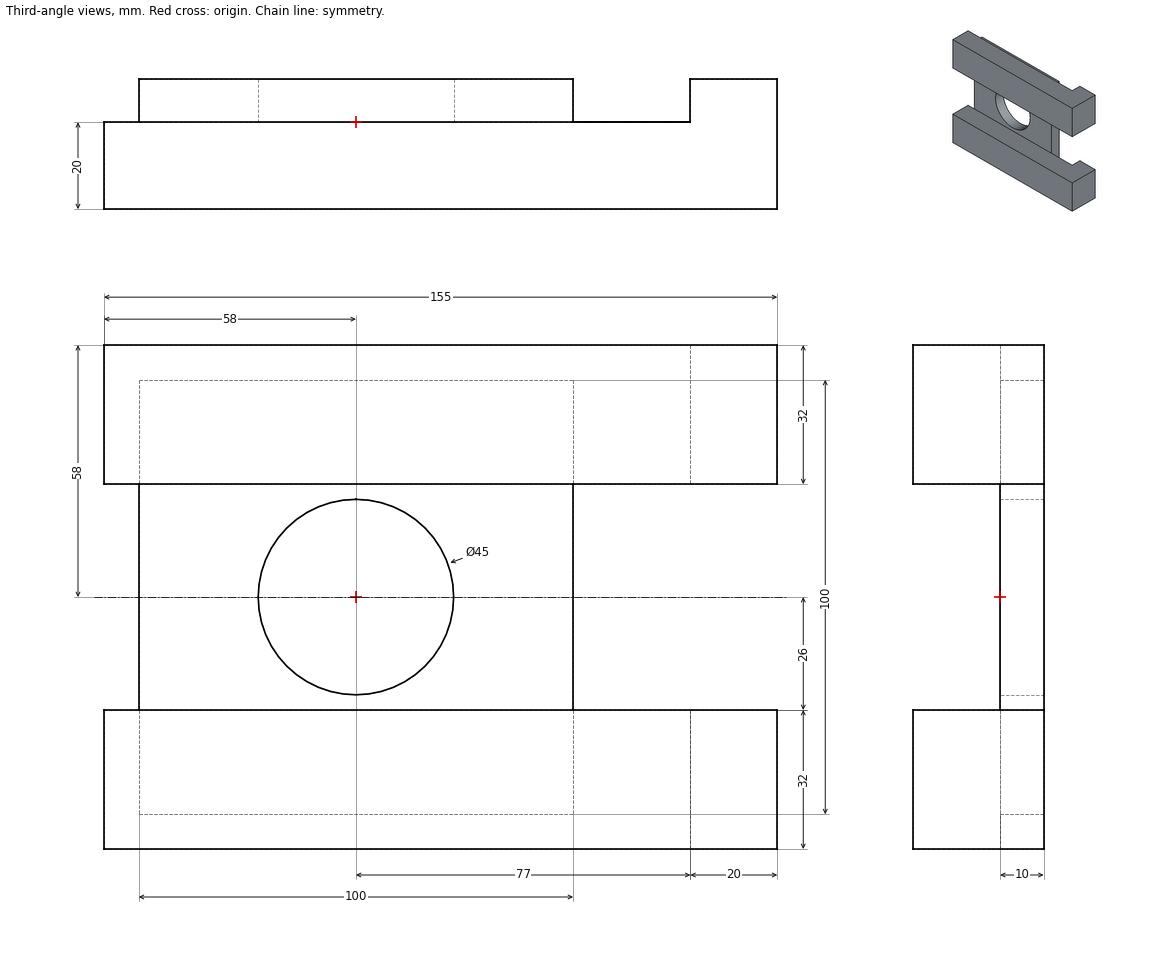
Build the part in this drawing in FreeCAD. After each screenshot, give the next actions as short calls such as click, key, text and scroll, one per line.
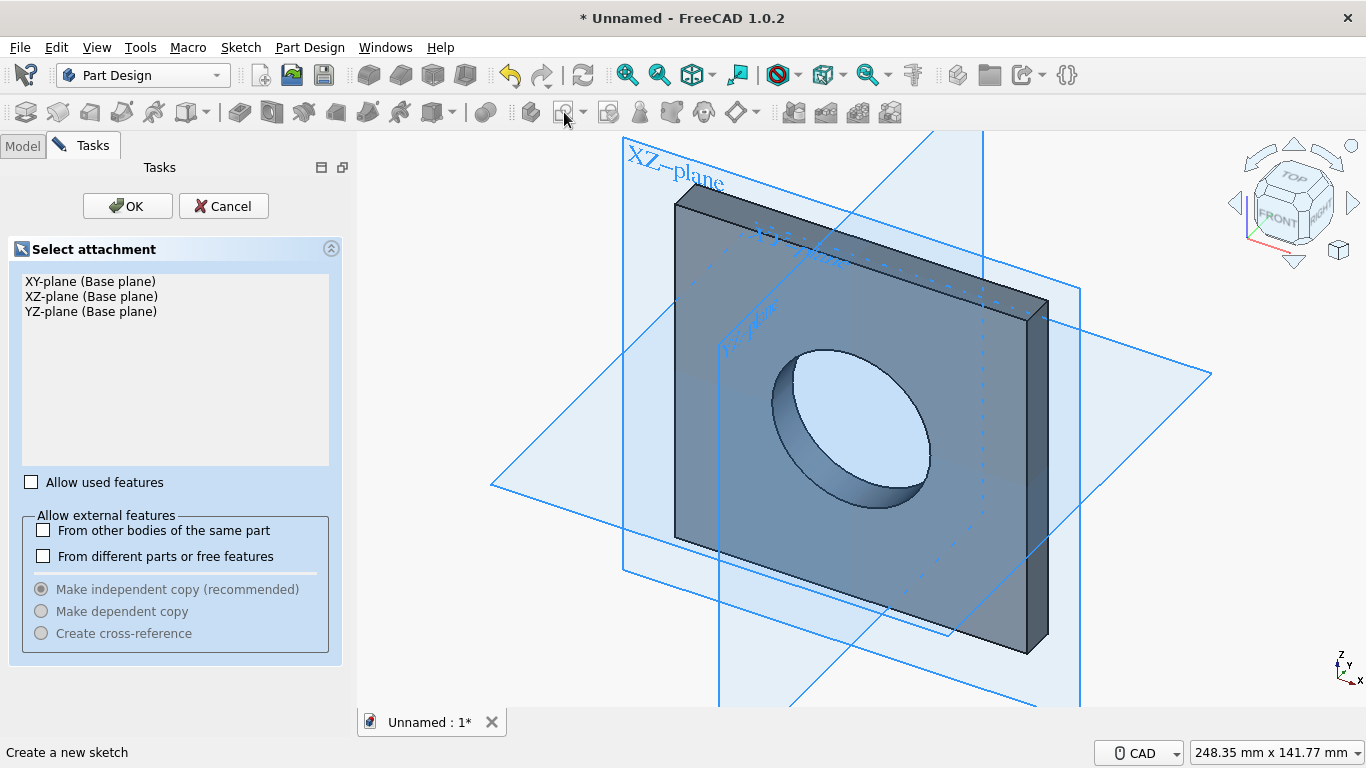
click(82, 296)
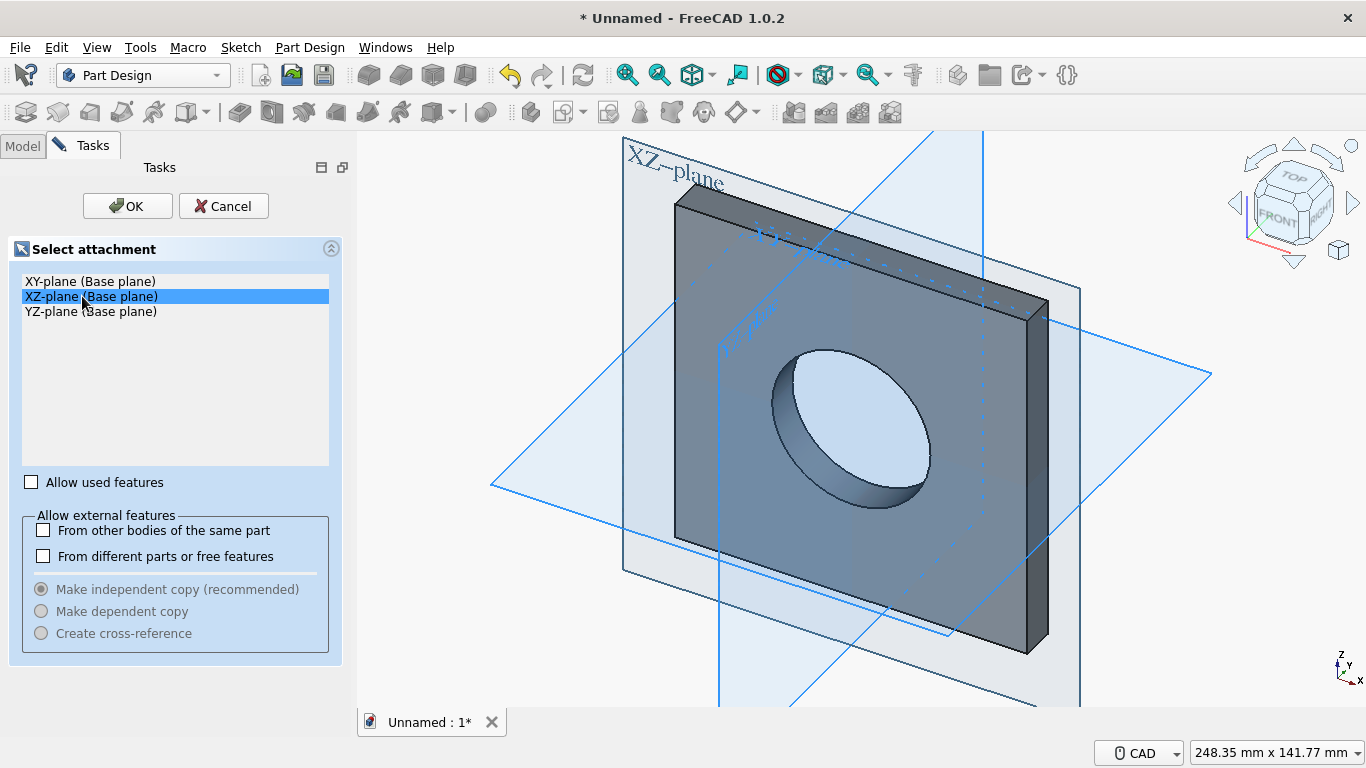
click(128, 206)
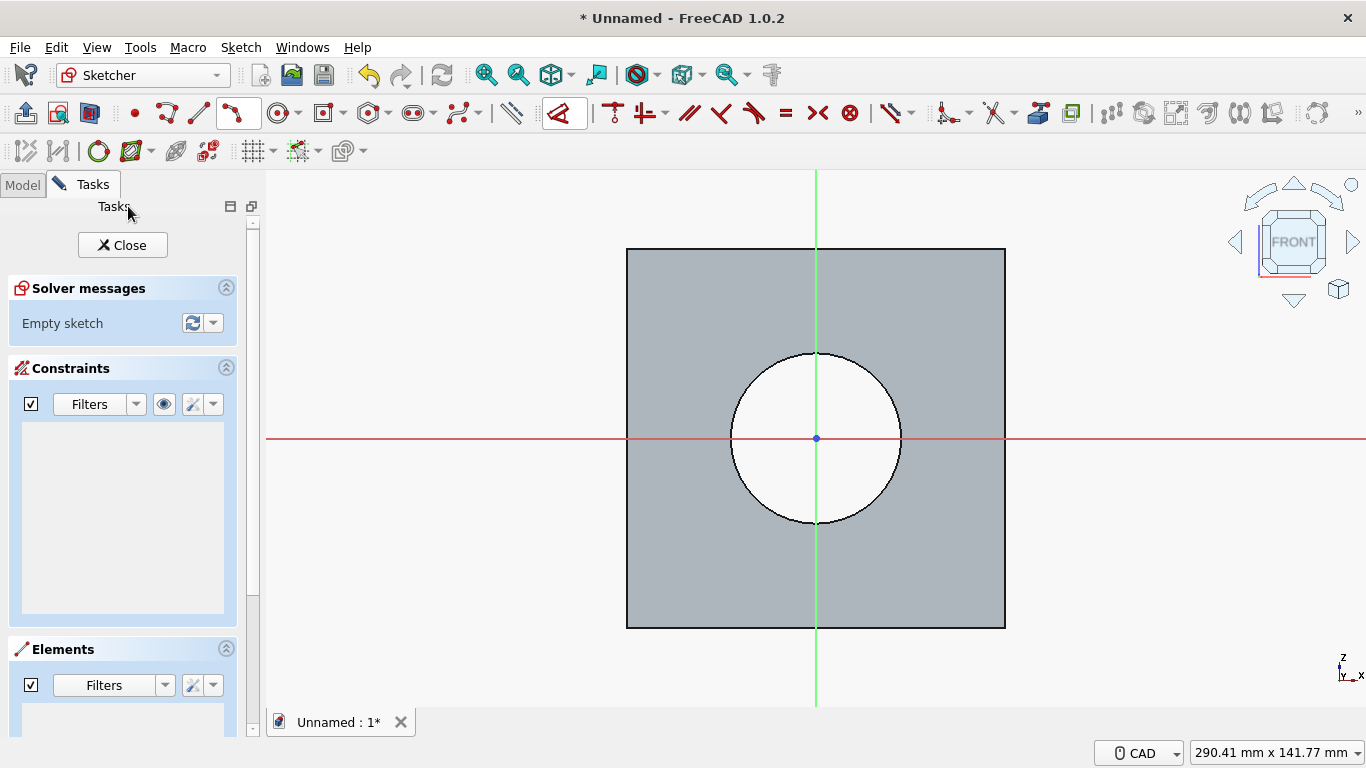
scroll(294, 439, down, 1)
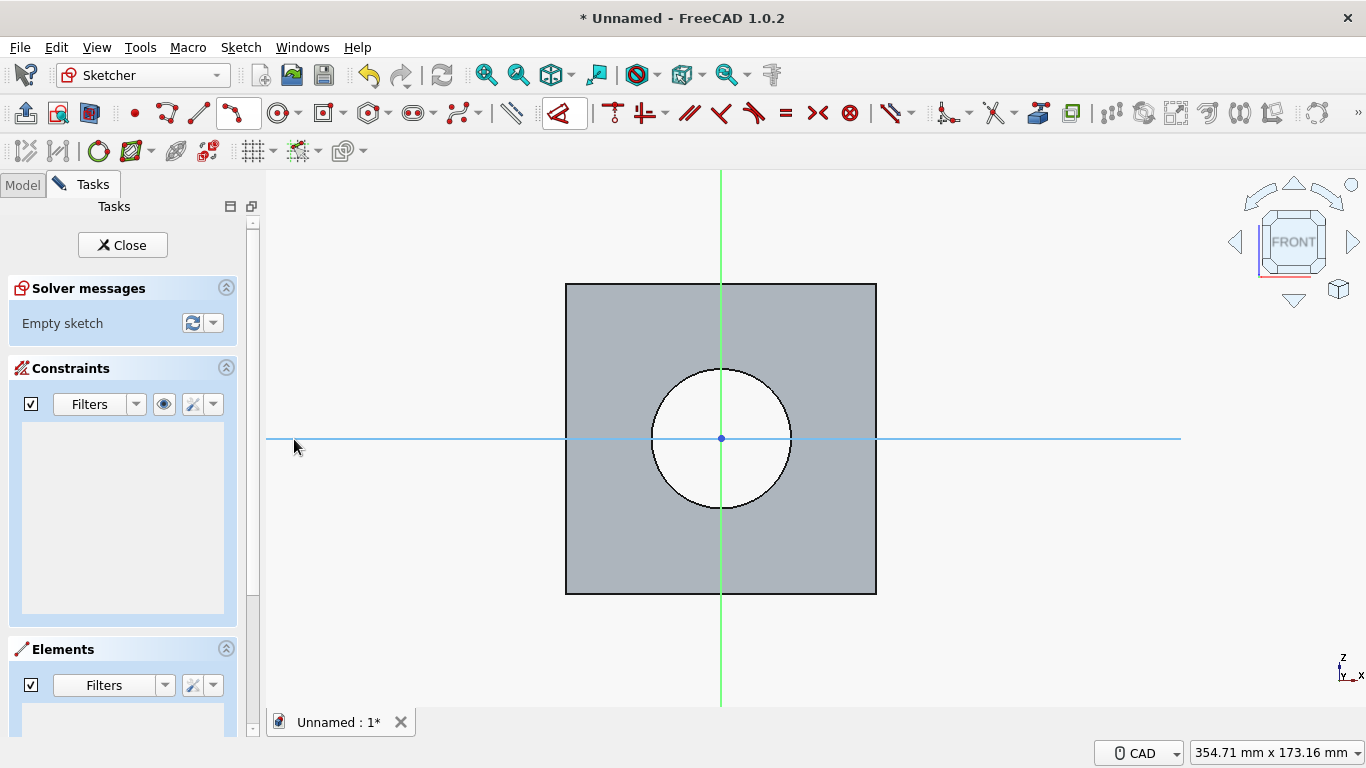
key(g)
key(r)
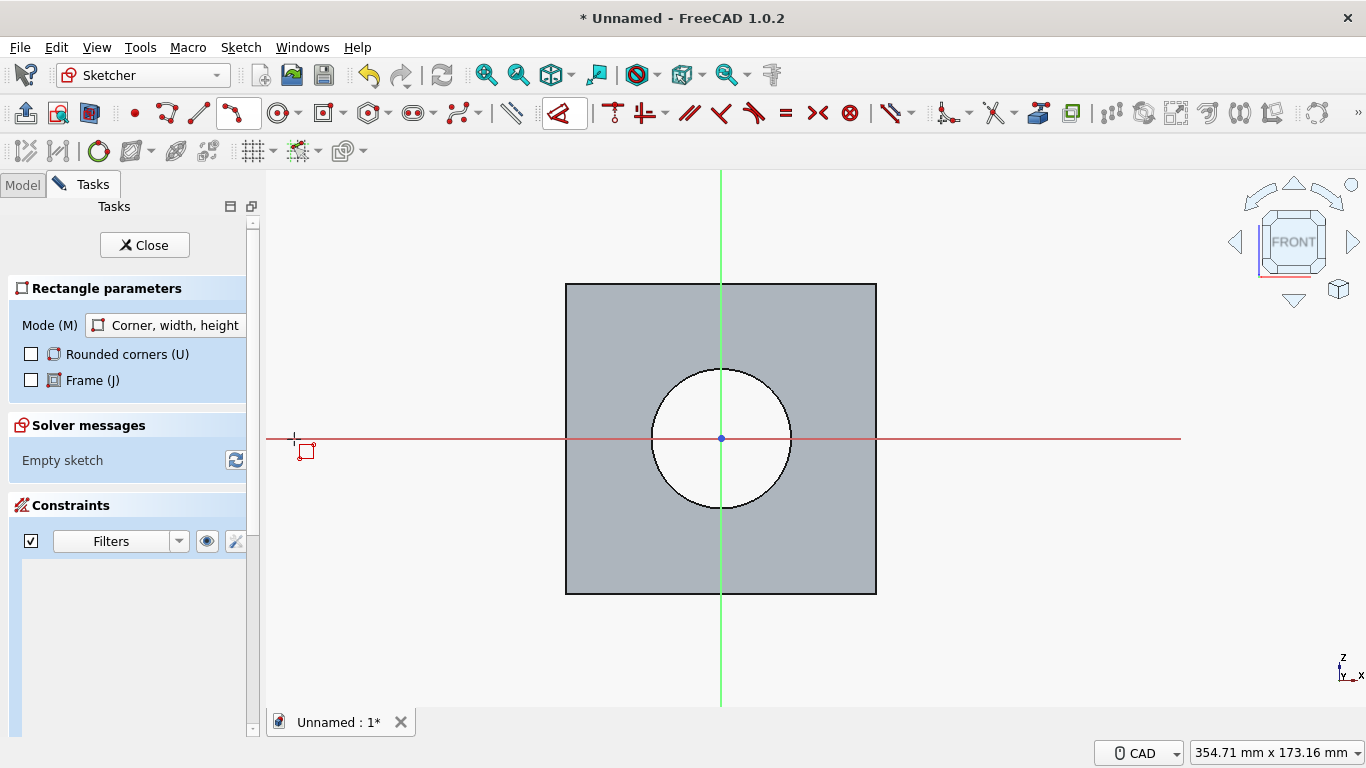
click(542, 259)
move(1022, 358)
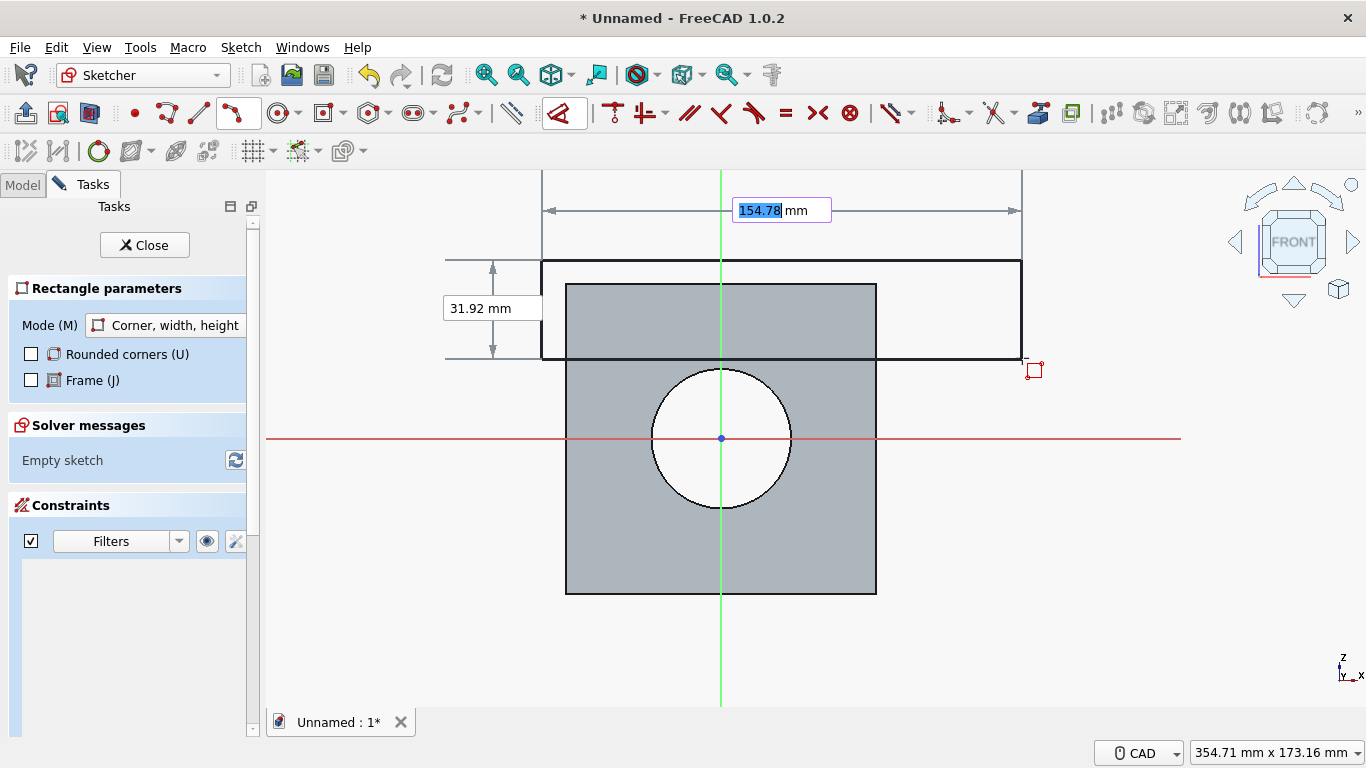
text(155)
key(Tab)
text(32)
key(Return)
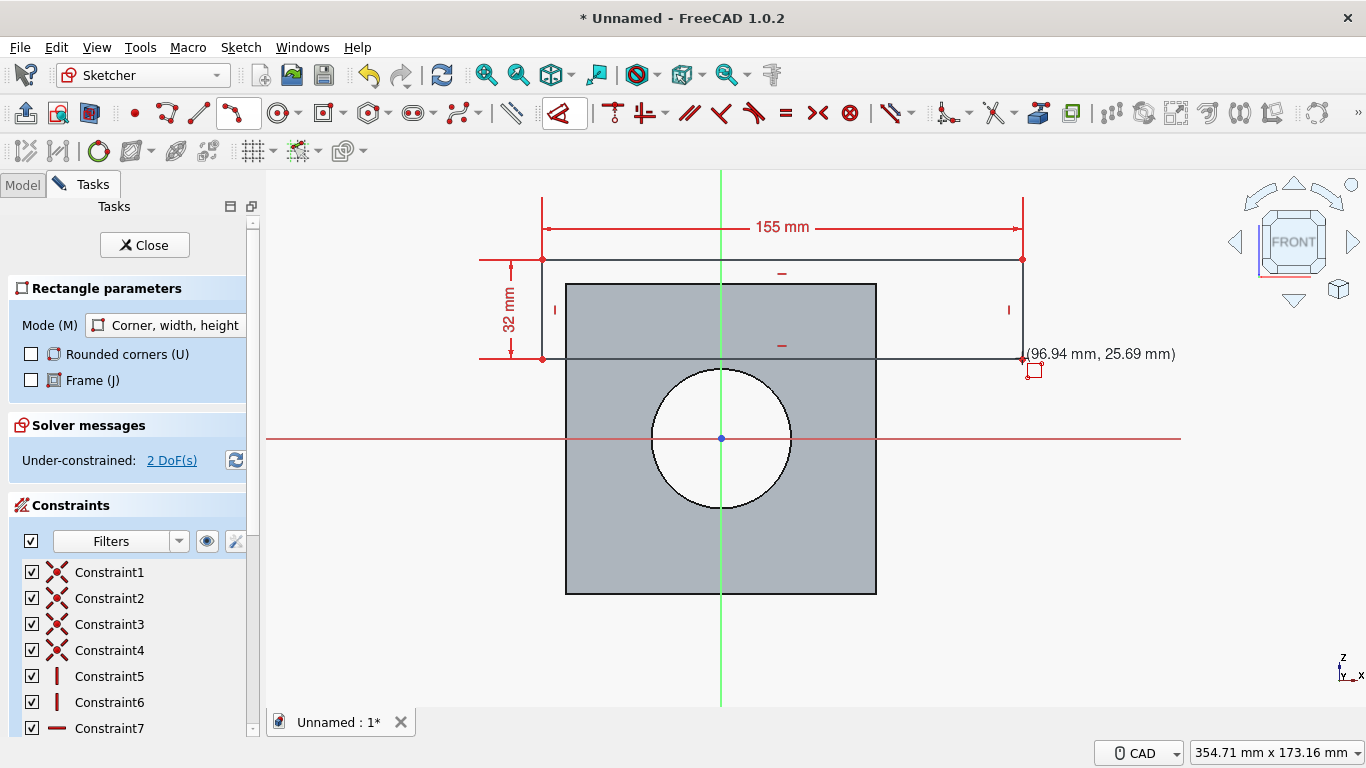
click(542, 519)
move(1022, 619)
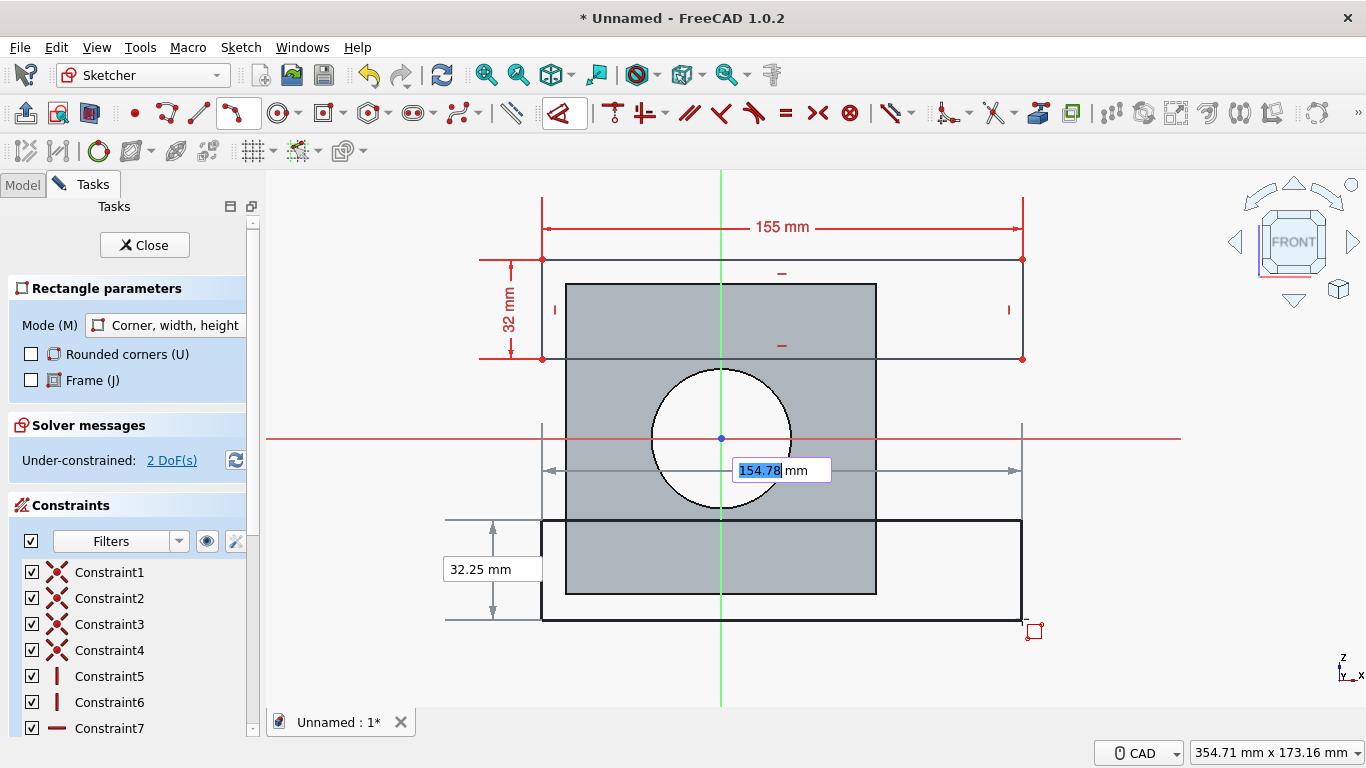
text(155)
key(Tab)
text(32)
key(Return)
key(Escape)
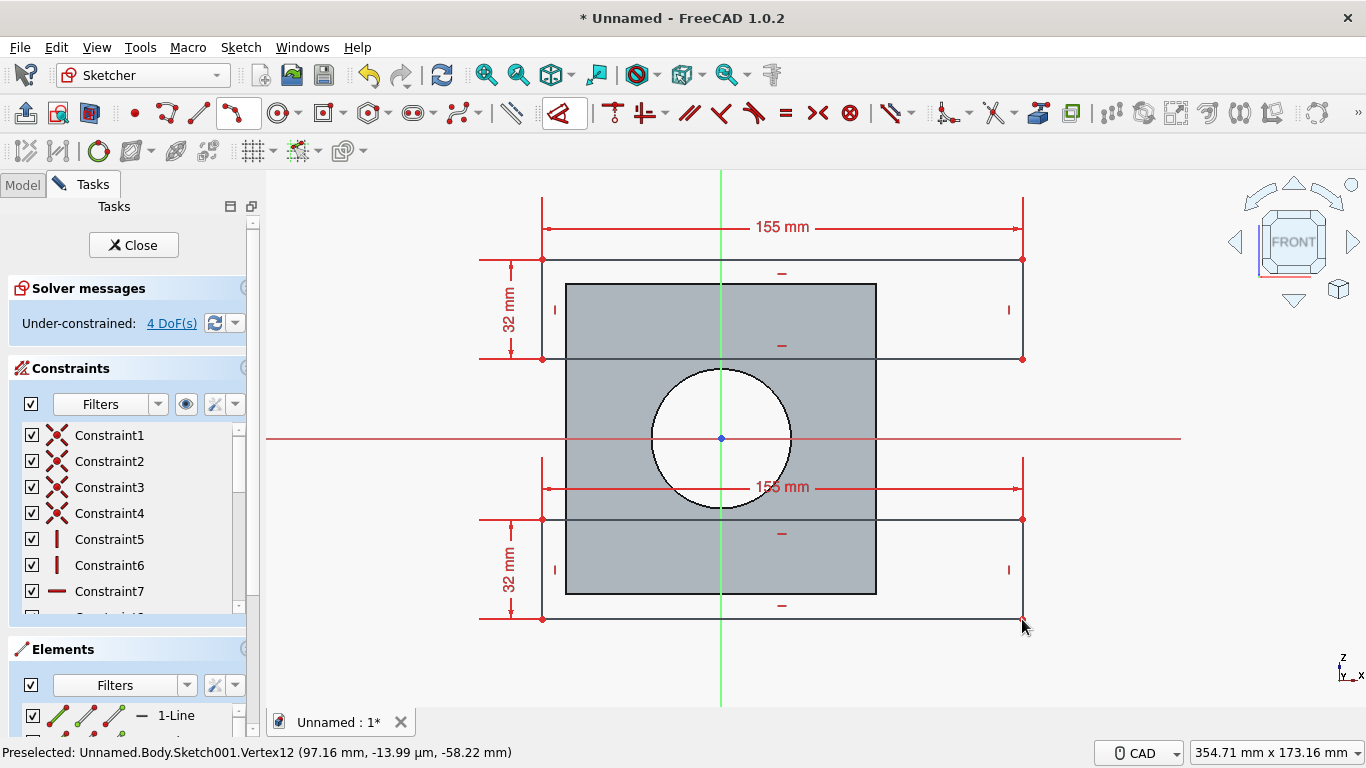
click(542, 359)